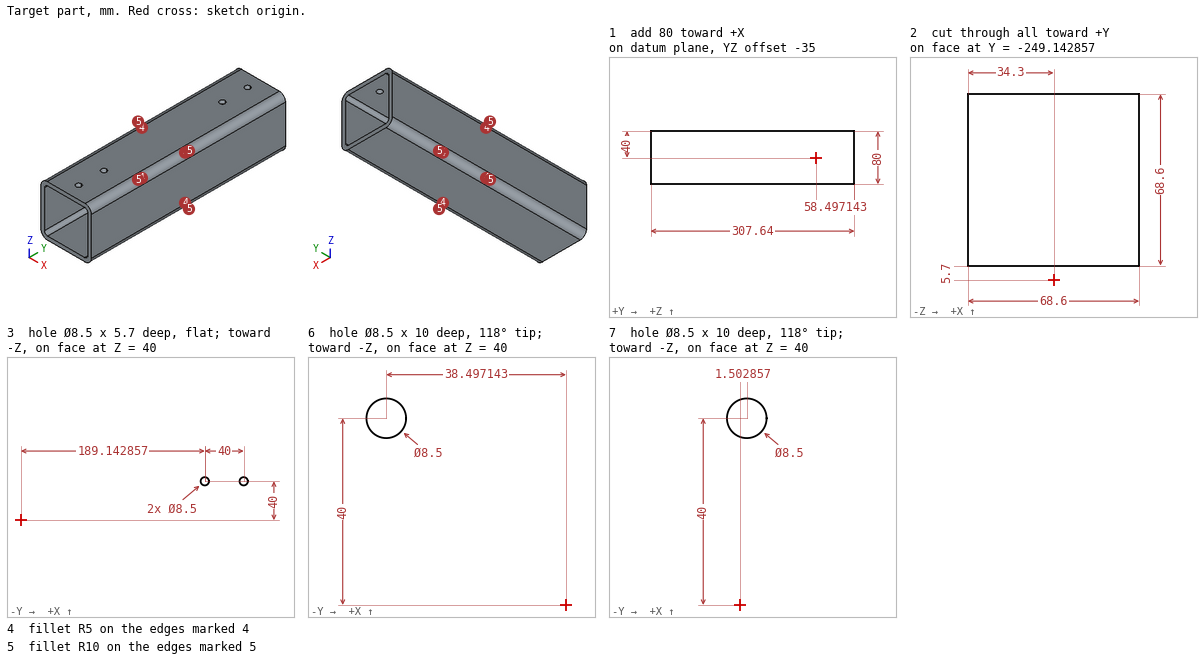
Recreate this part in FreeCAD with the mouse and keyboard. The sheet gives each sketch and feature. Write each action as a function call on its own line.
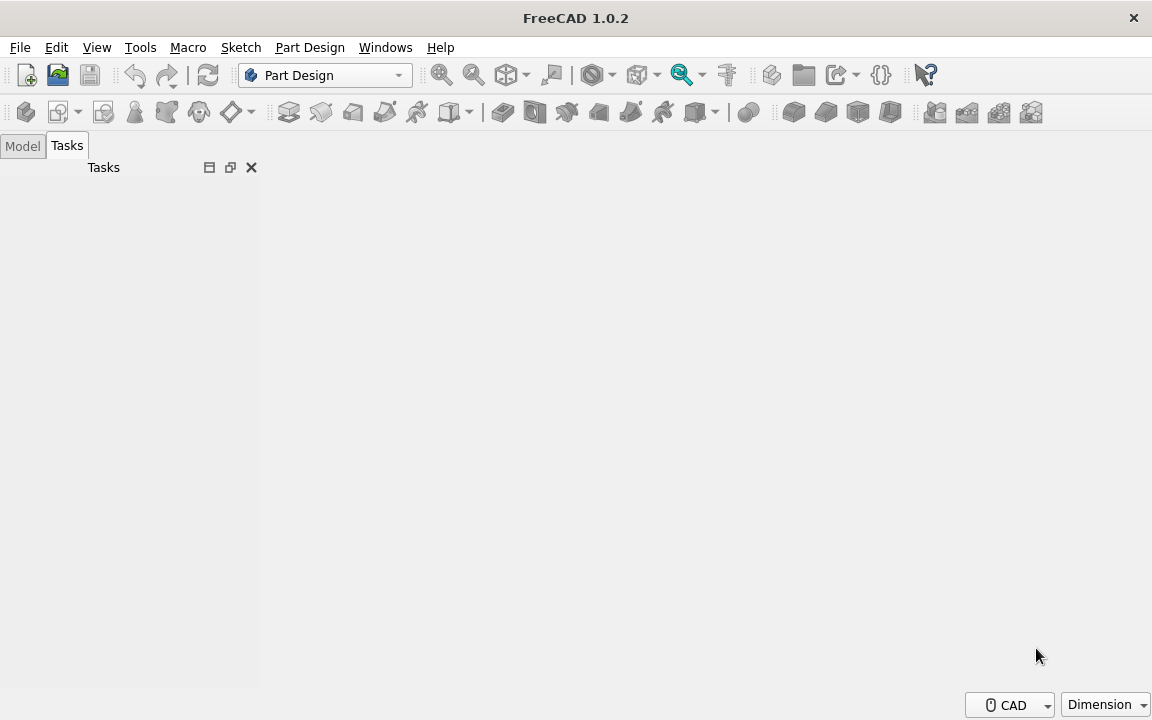
click(26, 76)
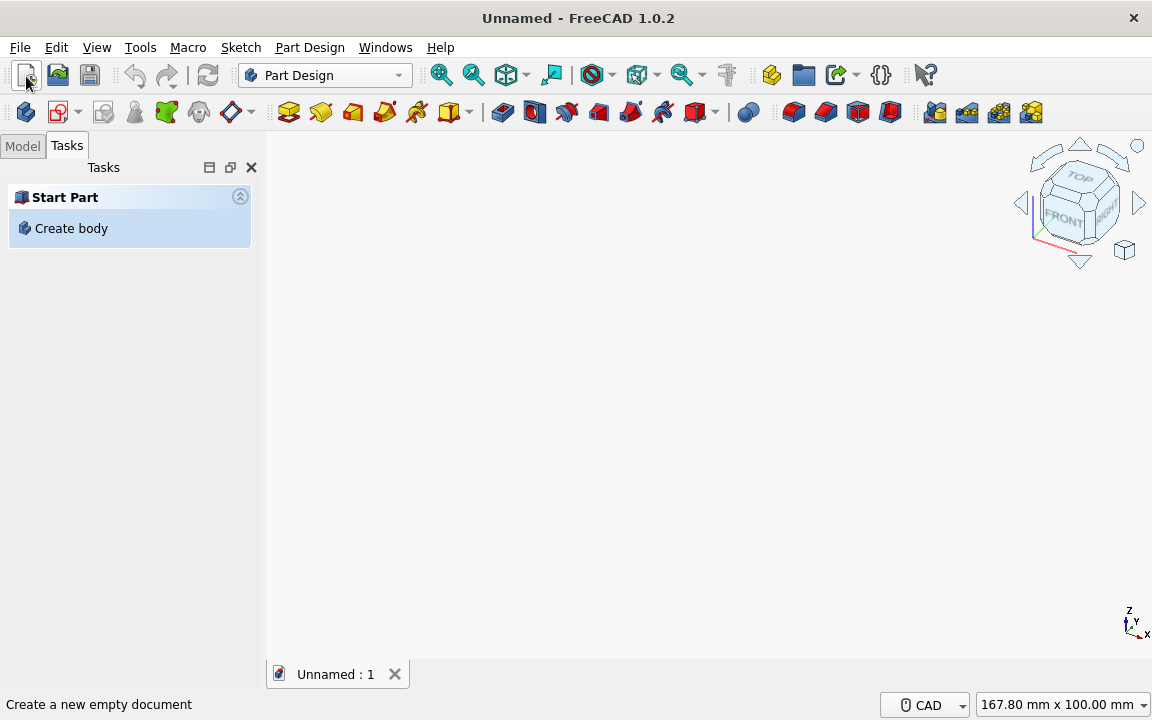
click(26, 112)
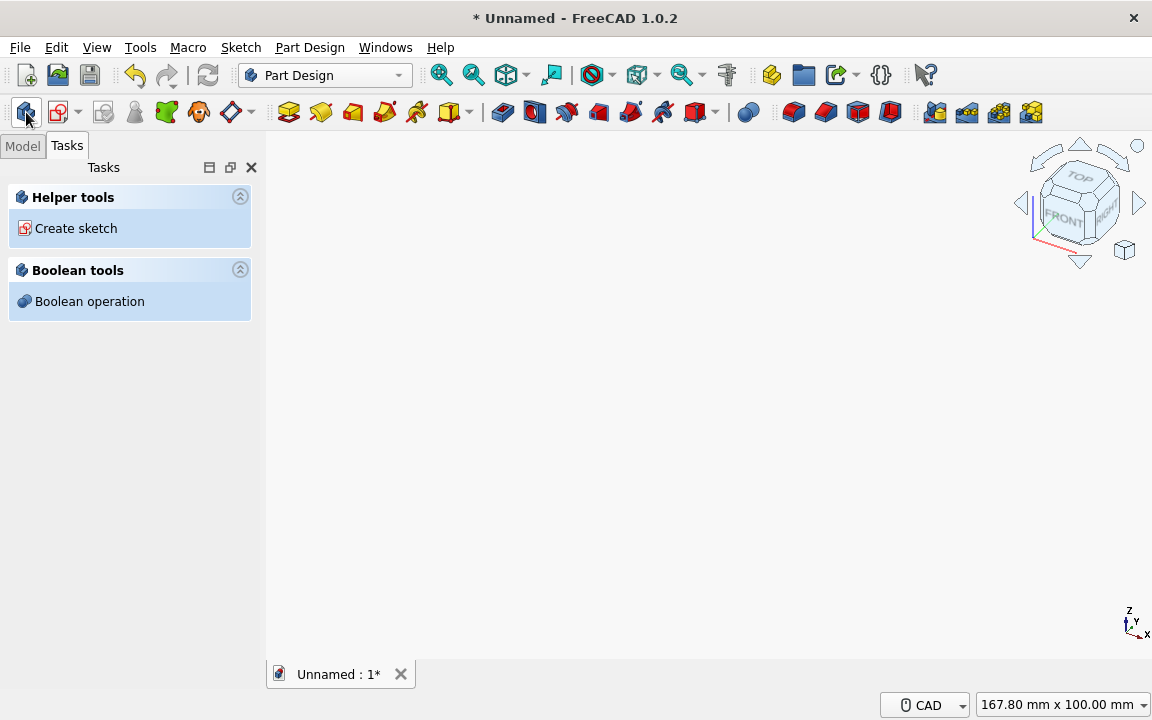
click(23, 145)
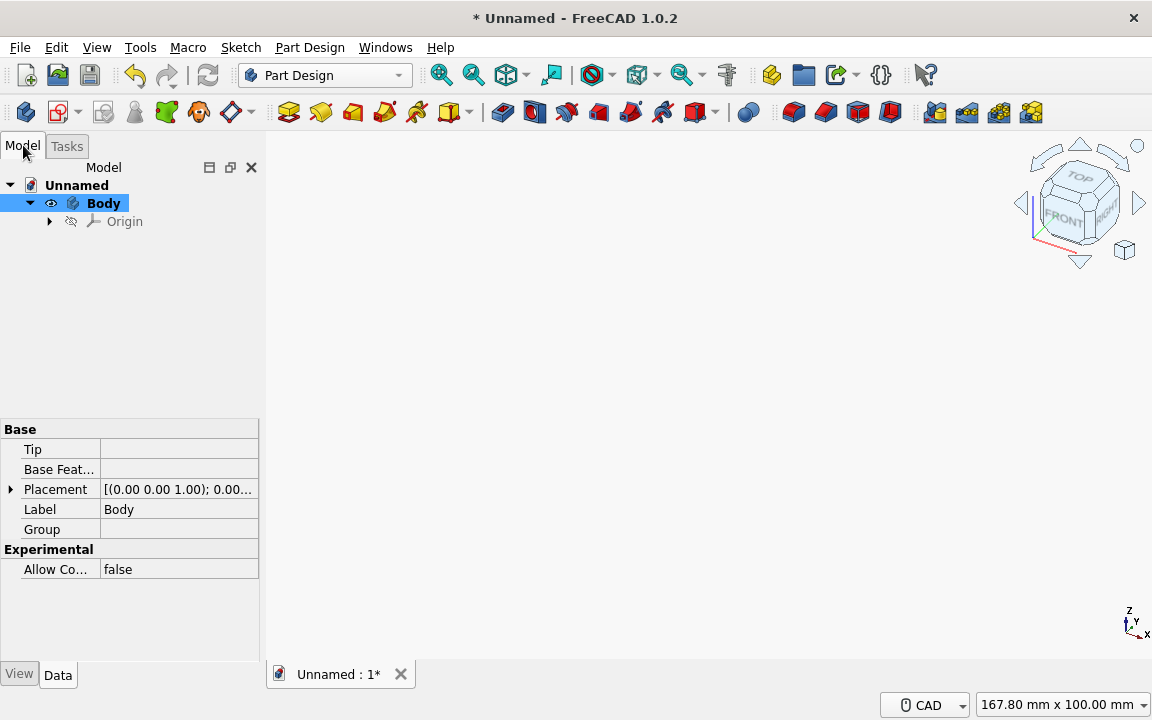
click(50, 221)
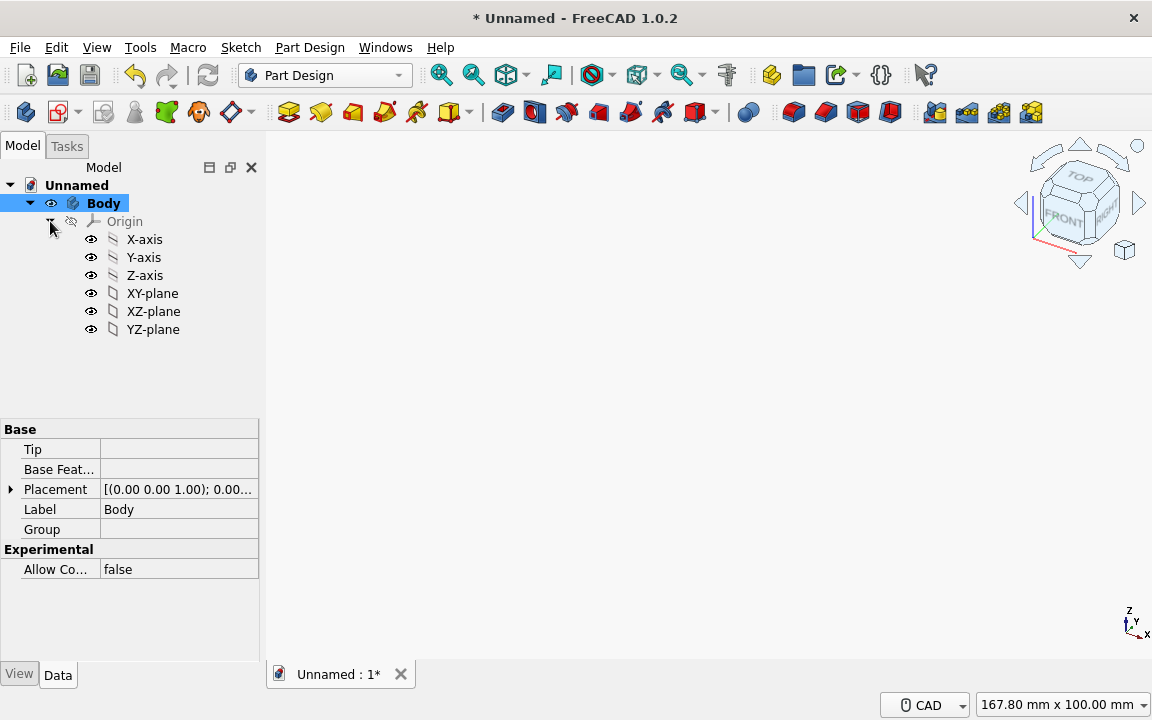
click(136, 329)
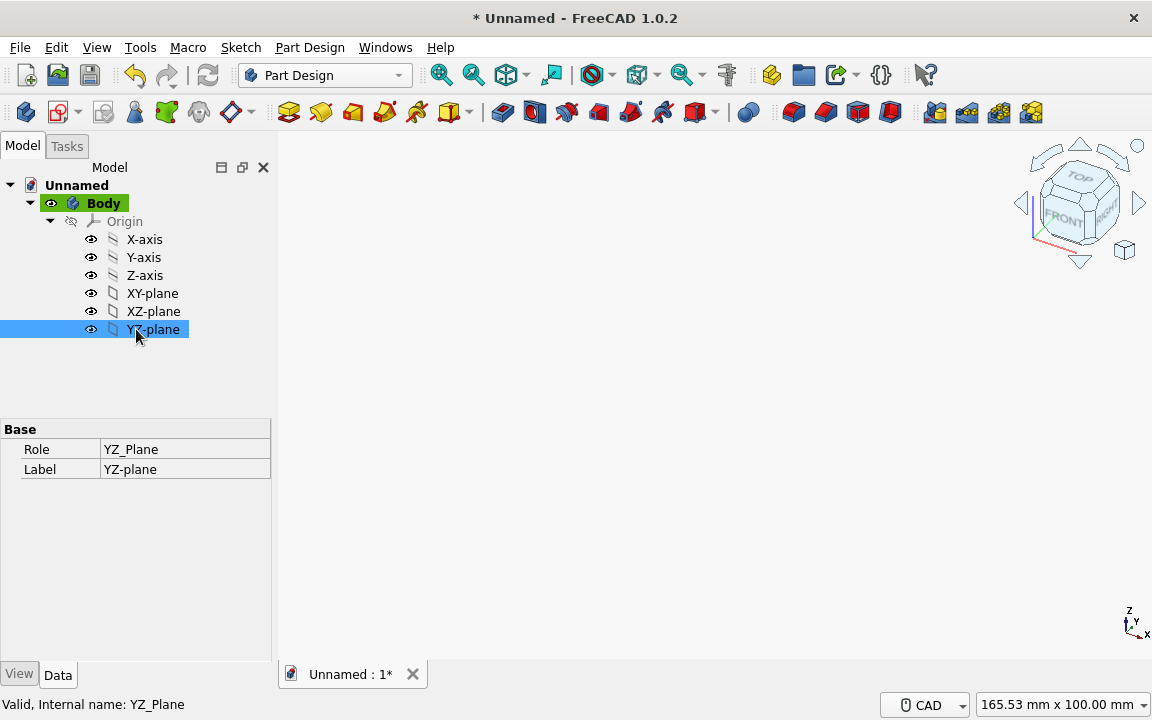
click(232, 112)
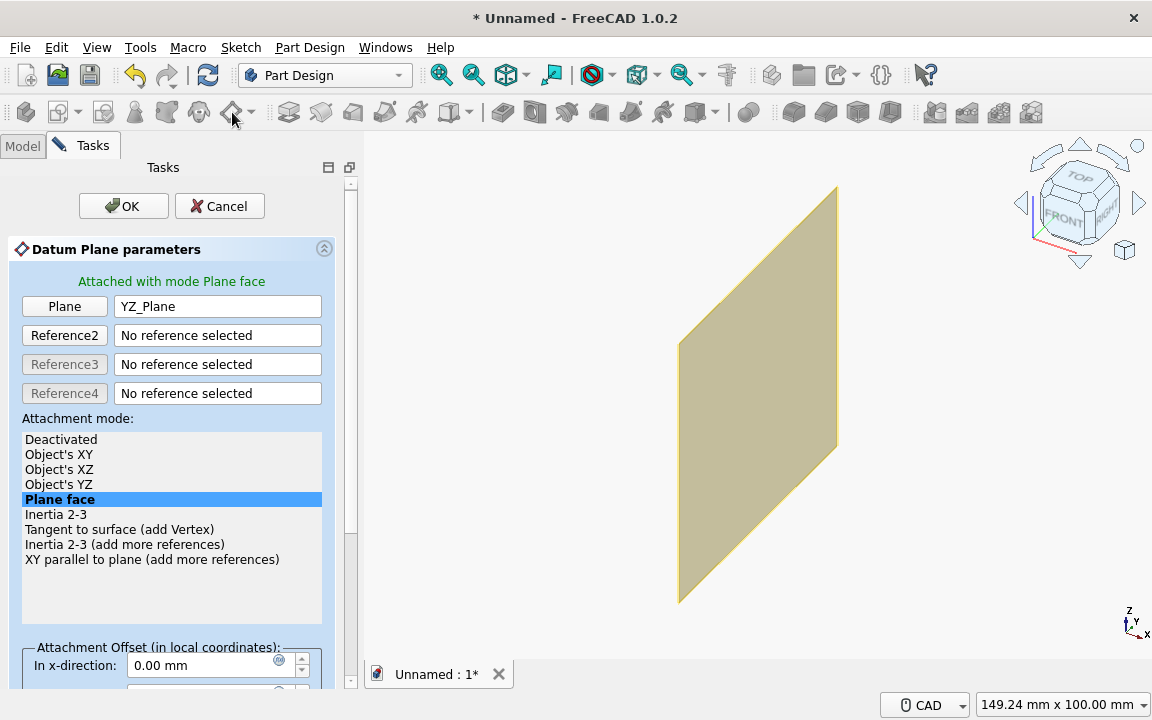
scroll(351, 432, down, 2)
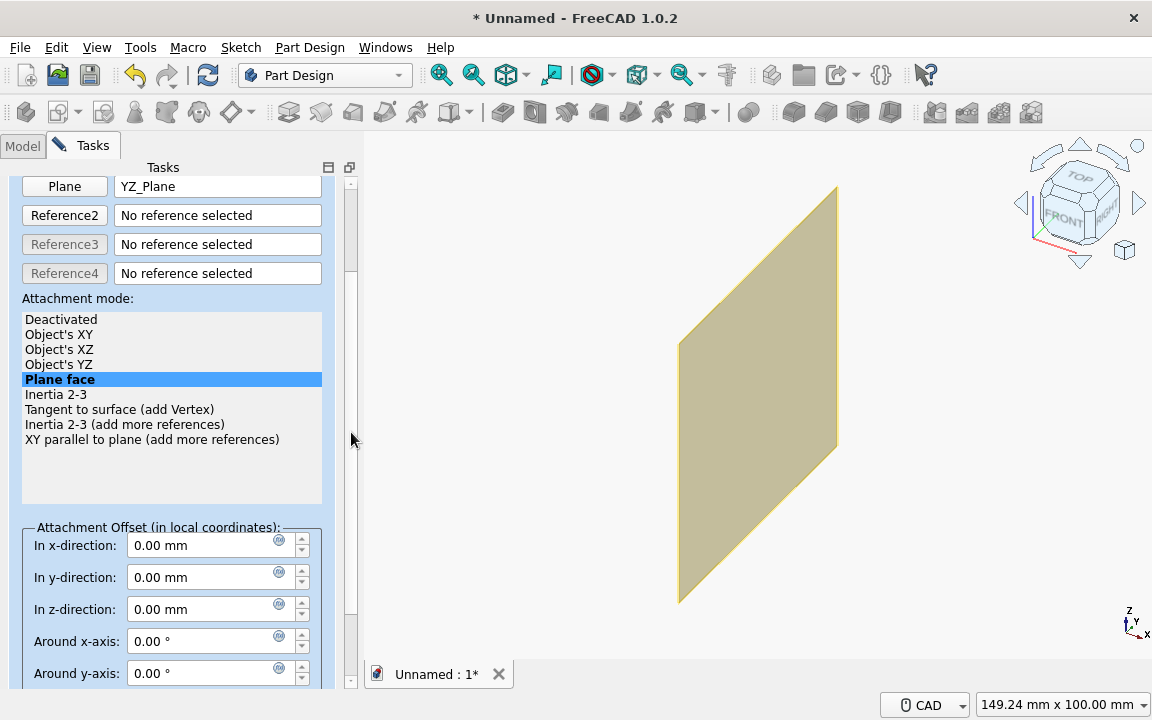
triple_click(210, 609)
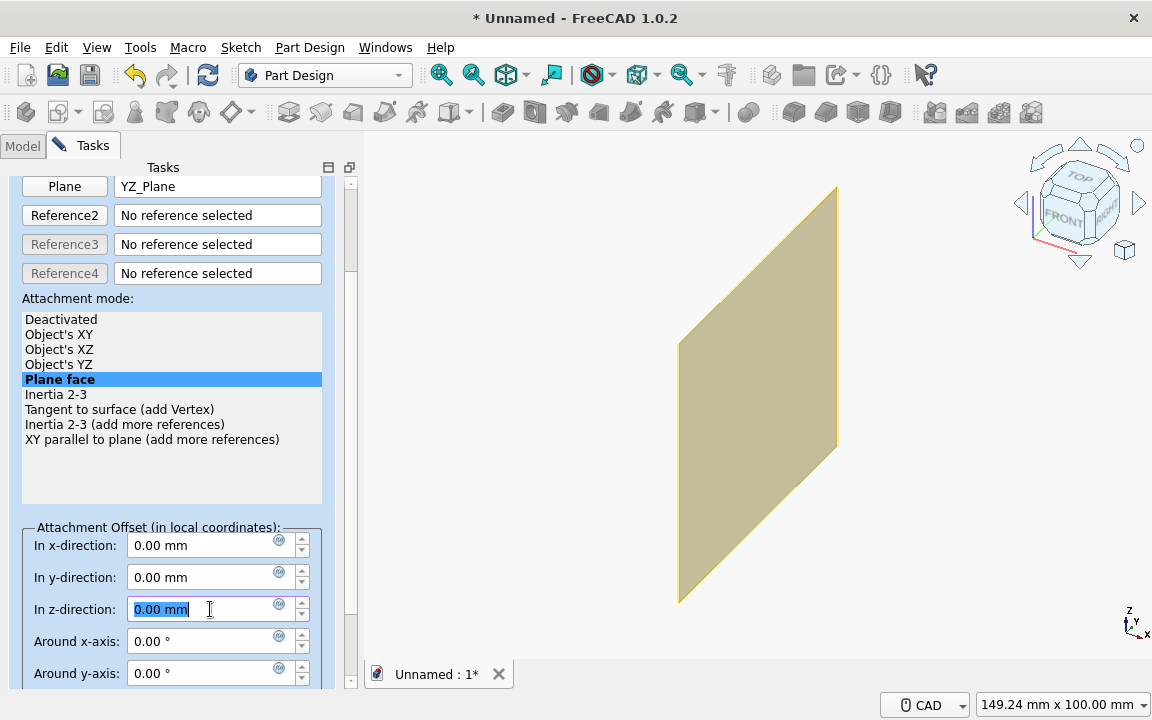
text(-35)
key(Tab)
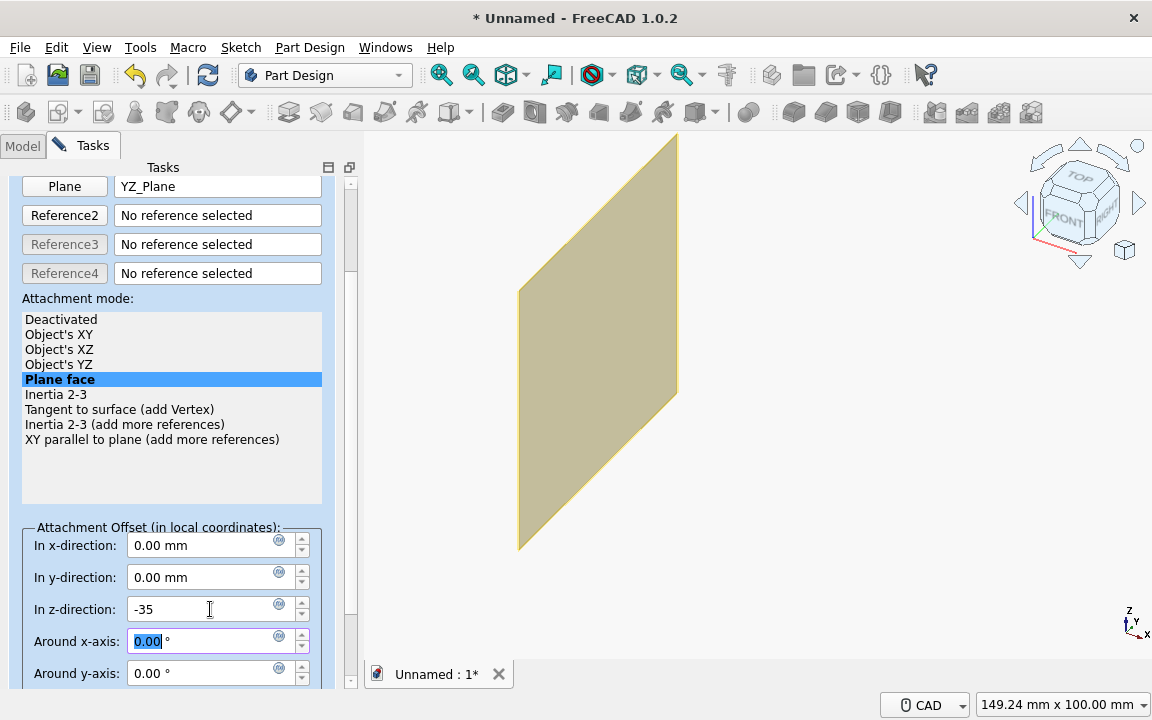
scroll(351, 432, up, 3)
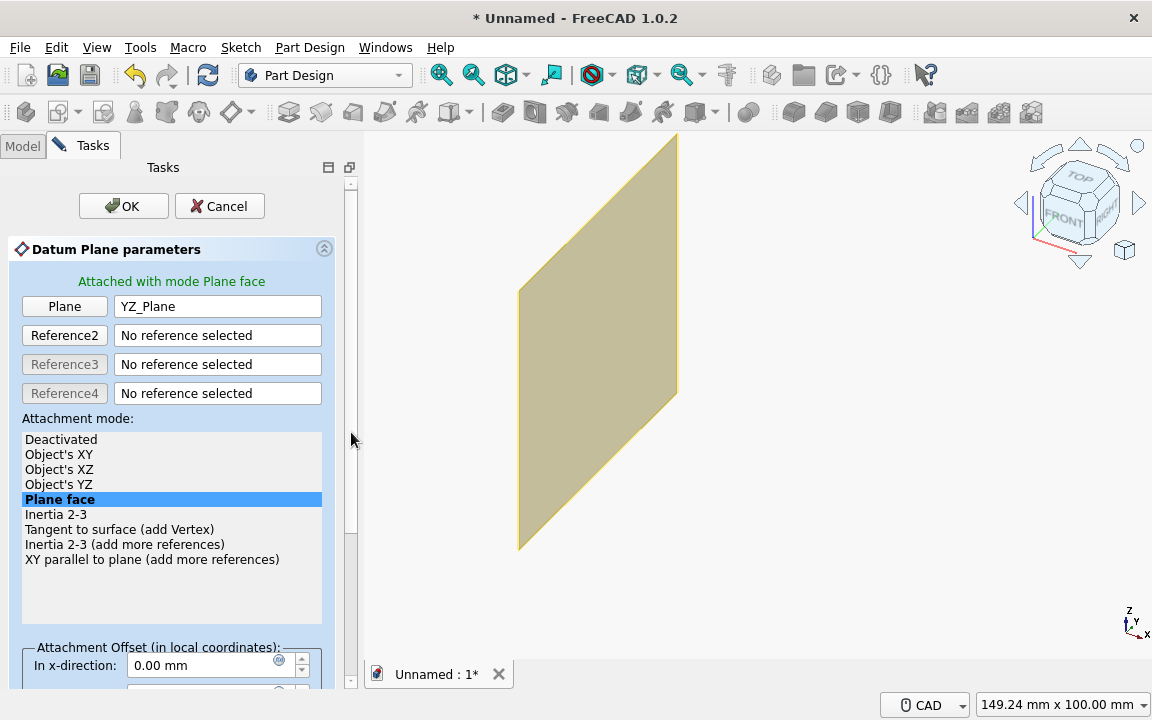
click(124, 206)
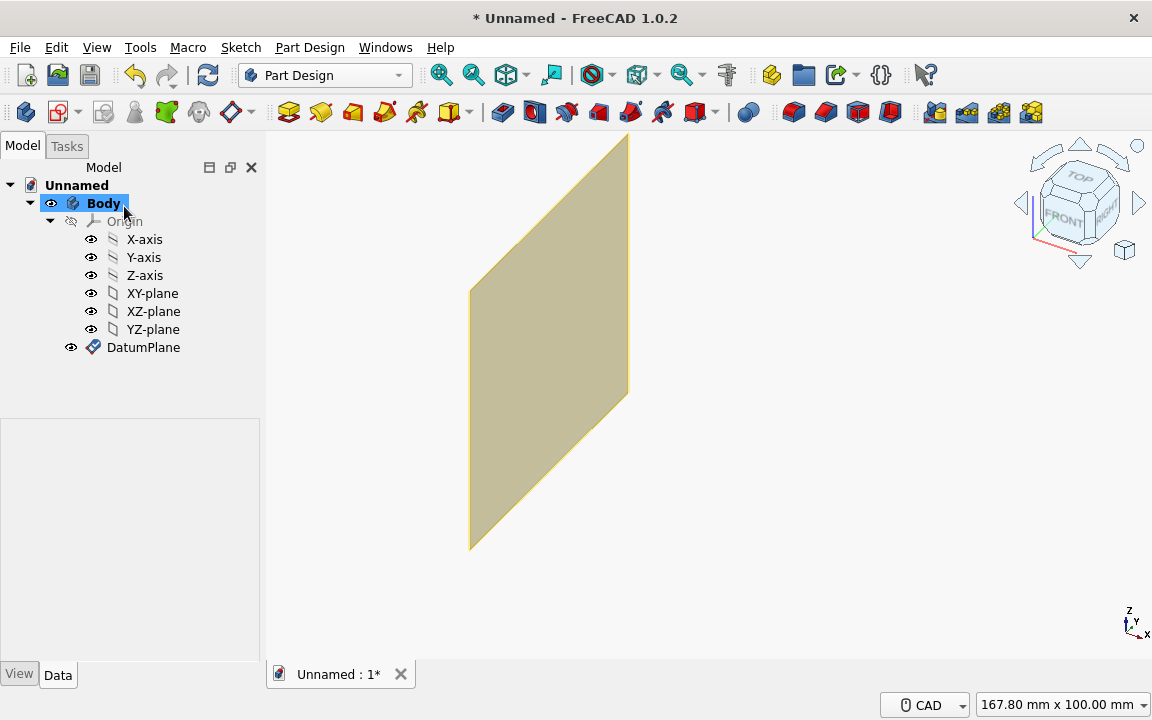
click(116, 347)